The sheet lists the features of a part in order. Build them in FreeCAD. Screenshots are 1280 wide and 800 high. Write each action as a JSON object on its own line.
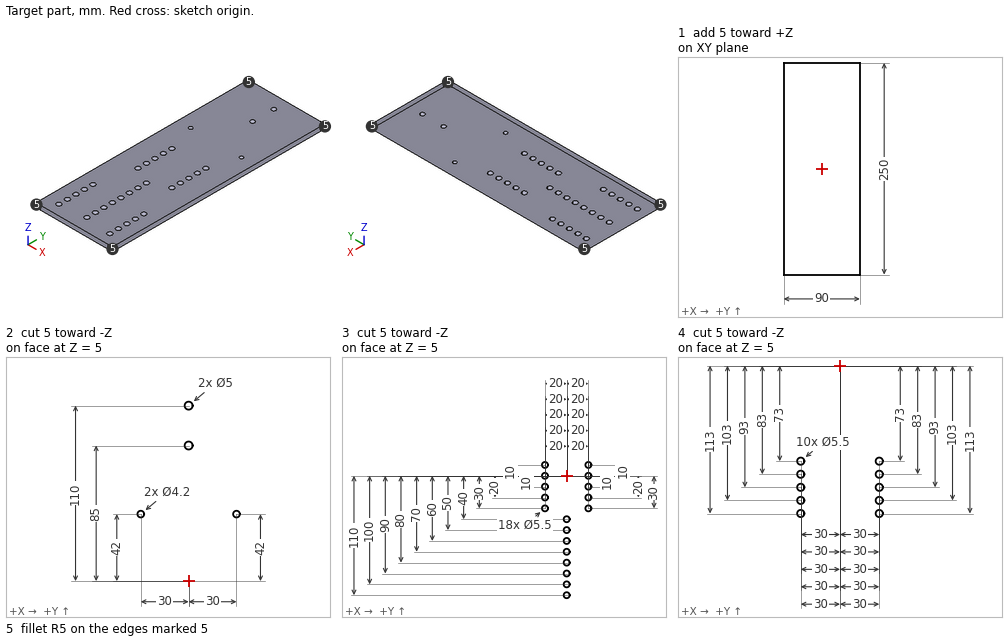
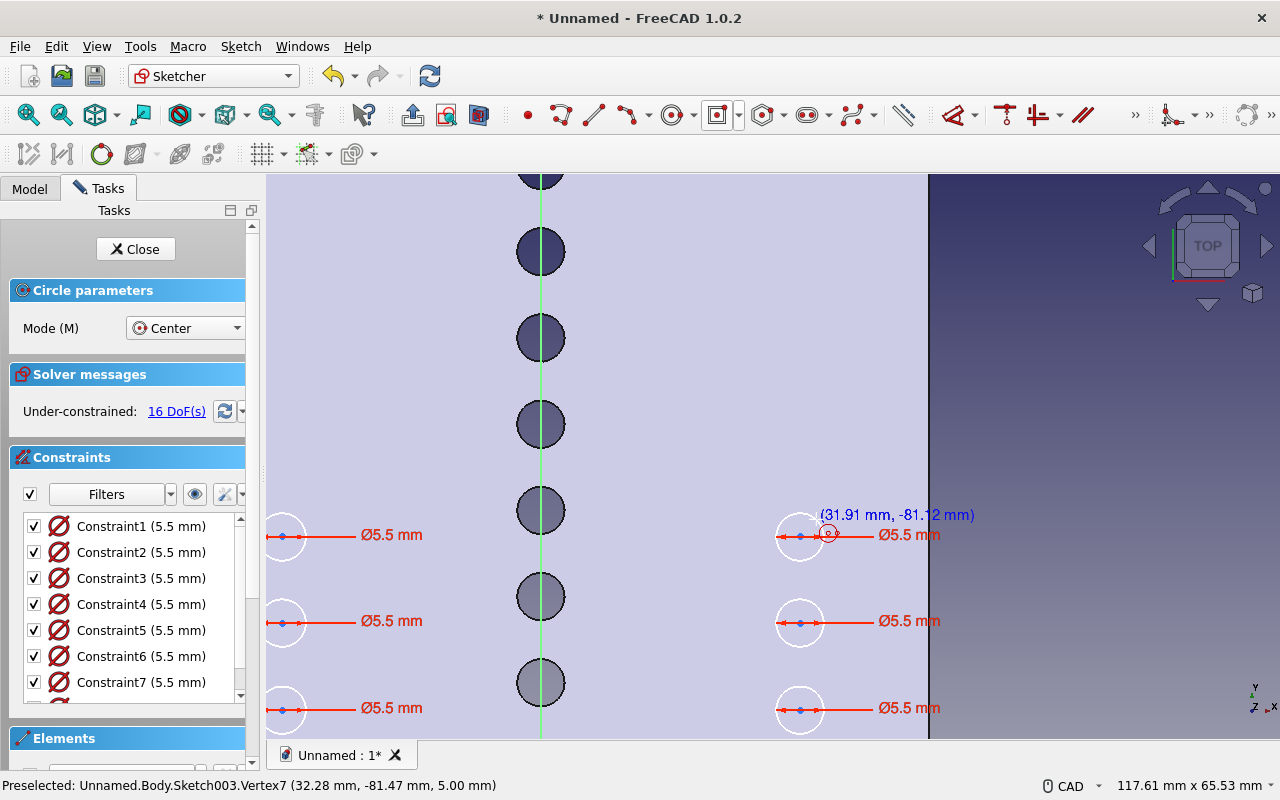
{"action": "scroll", "coordinate": [800, 536], "scroll_direction": "down", "scroll_amount": 5}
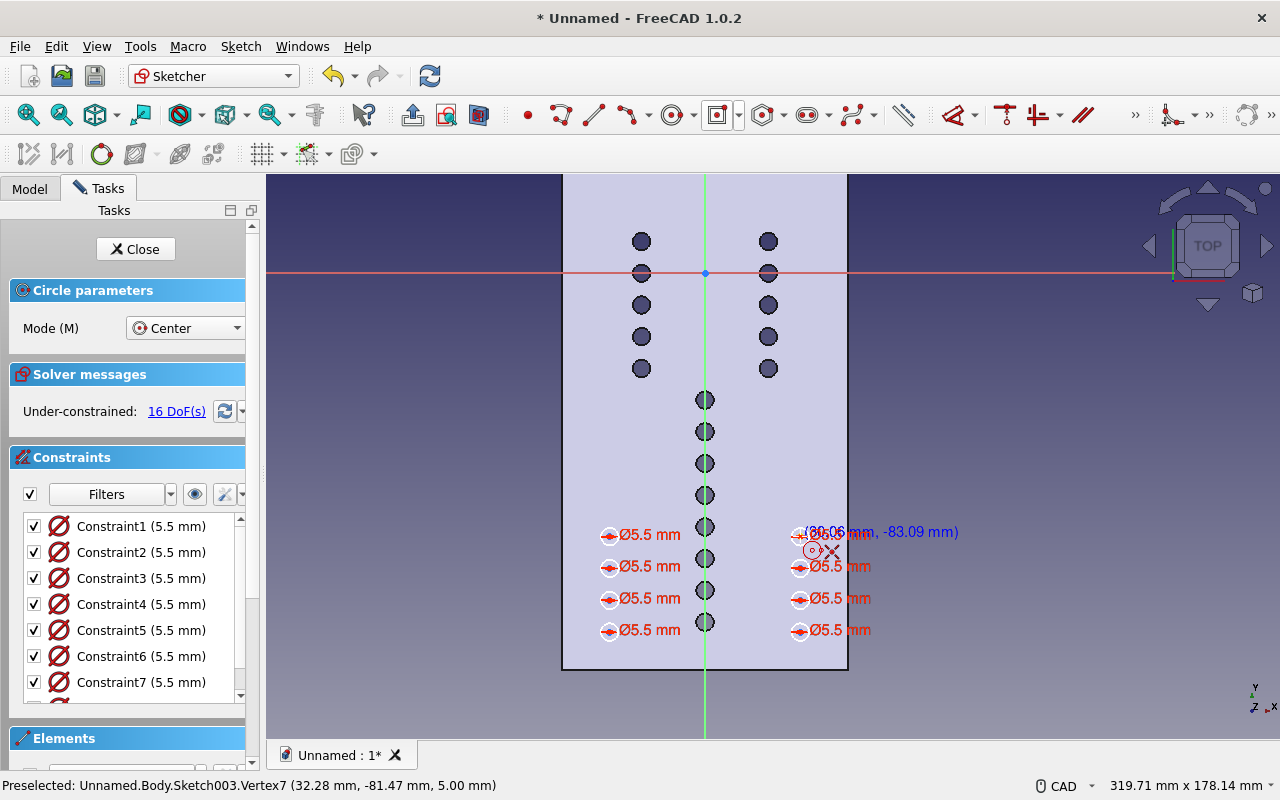
{"action": "scroll", "coordinate": [610, 505], "scroll_direction": "up", "scroll_amount": 5}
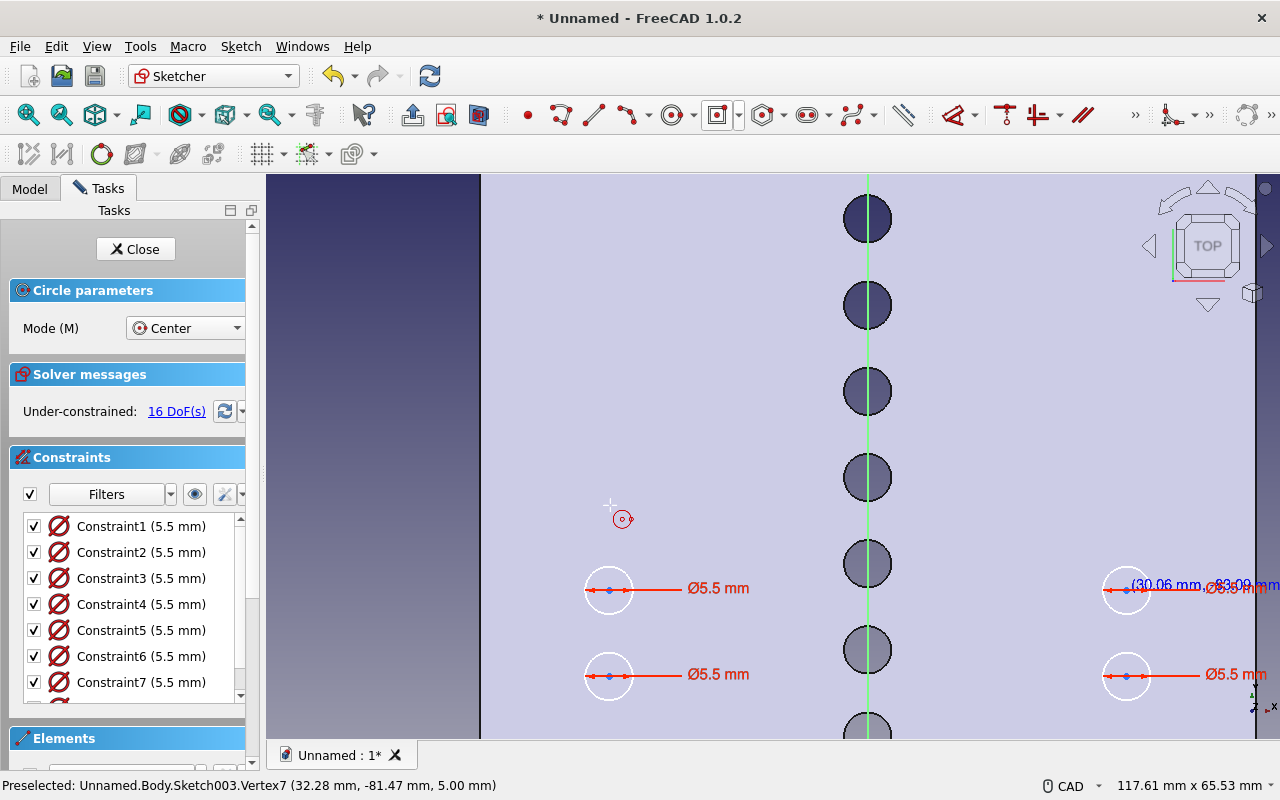
{"action": "left_click", "coordinate": [609, 503]}
{"action": "mouse_move", "coordinate": [626, 487]}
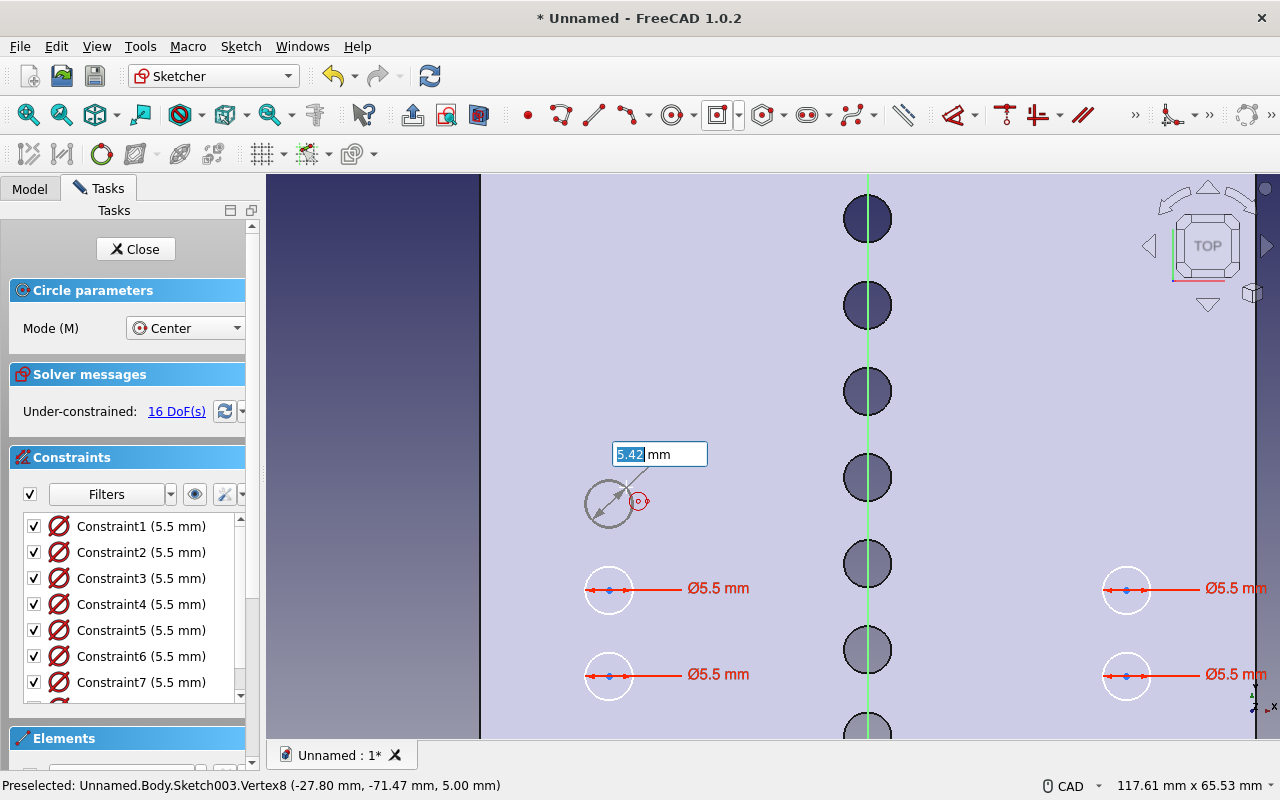
{"action": "type", "text": "5.5"}
{"action": "key", "text": "Return"}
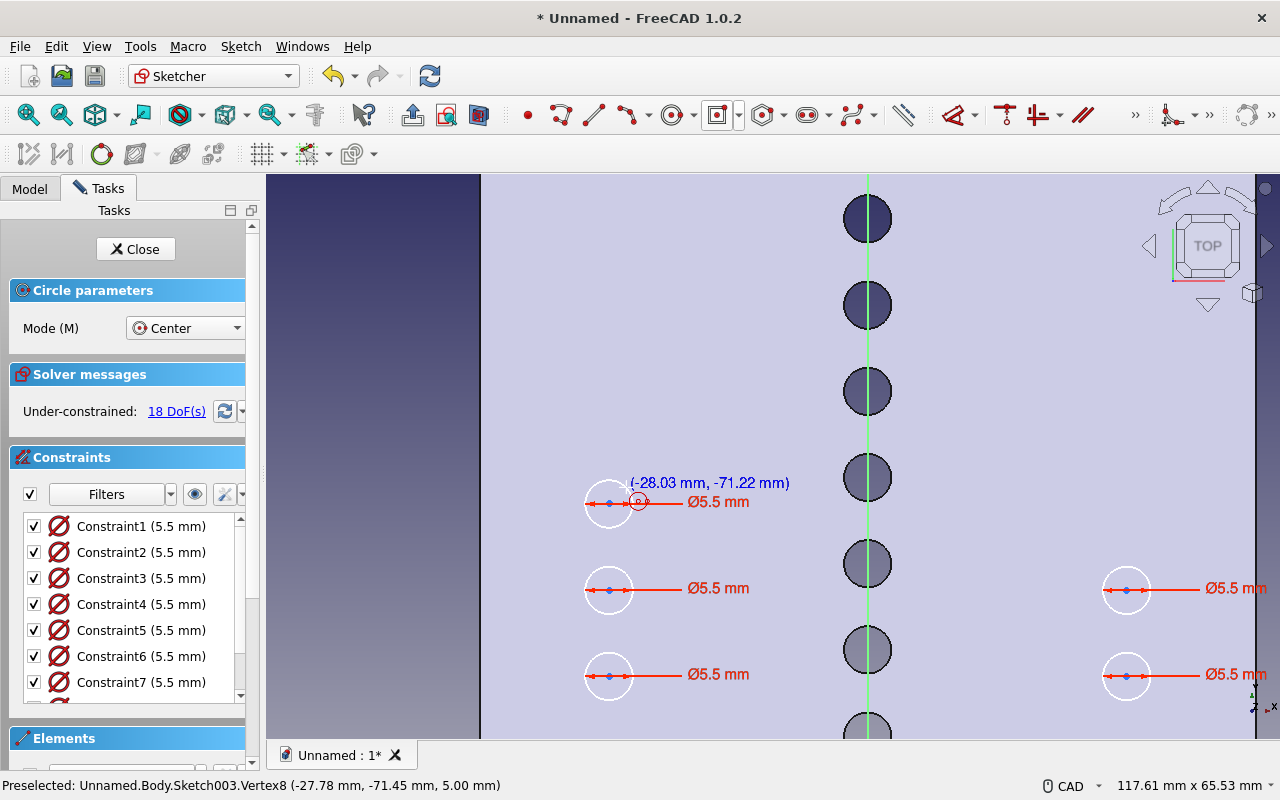
{"action": "scroll", "coordinate": [610, 505], "scroll_direction": "down", "scroll_amount": 5}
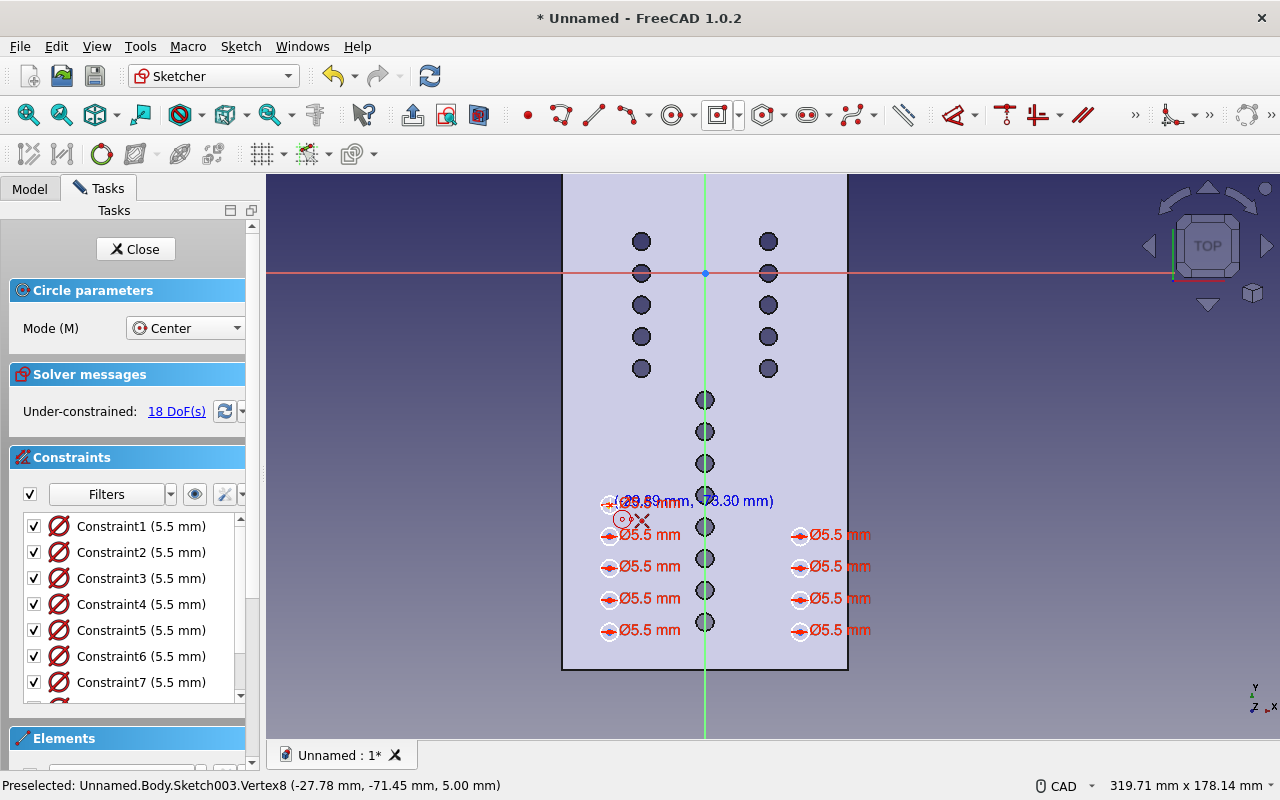
{"action": "scroll", "coordinate": [800, 505], "scroll_direction": "up", "scroll_amount": 5}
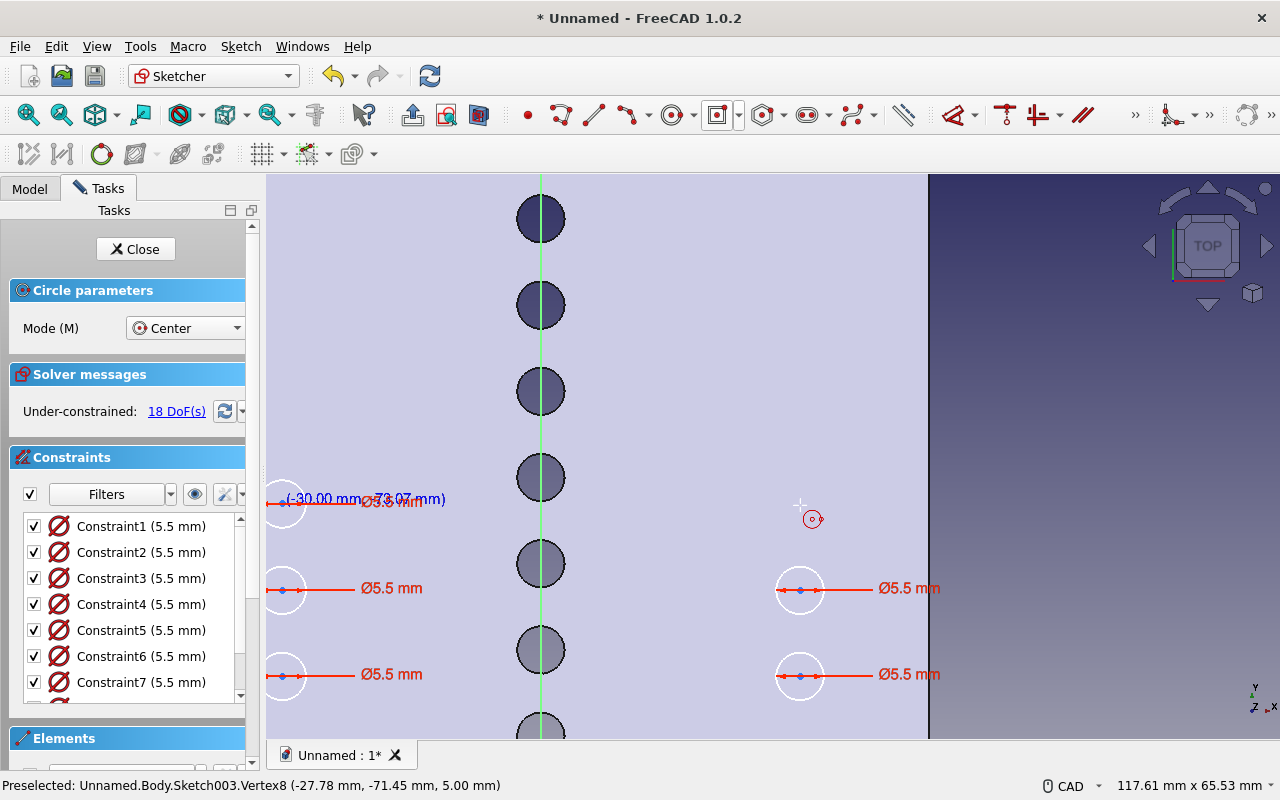
{"action": "left_click", "coordinate": [800, 503]}
{"action": "mouse_move", "coordinate": [816, 487]}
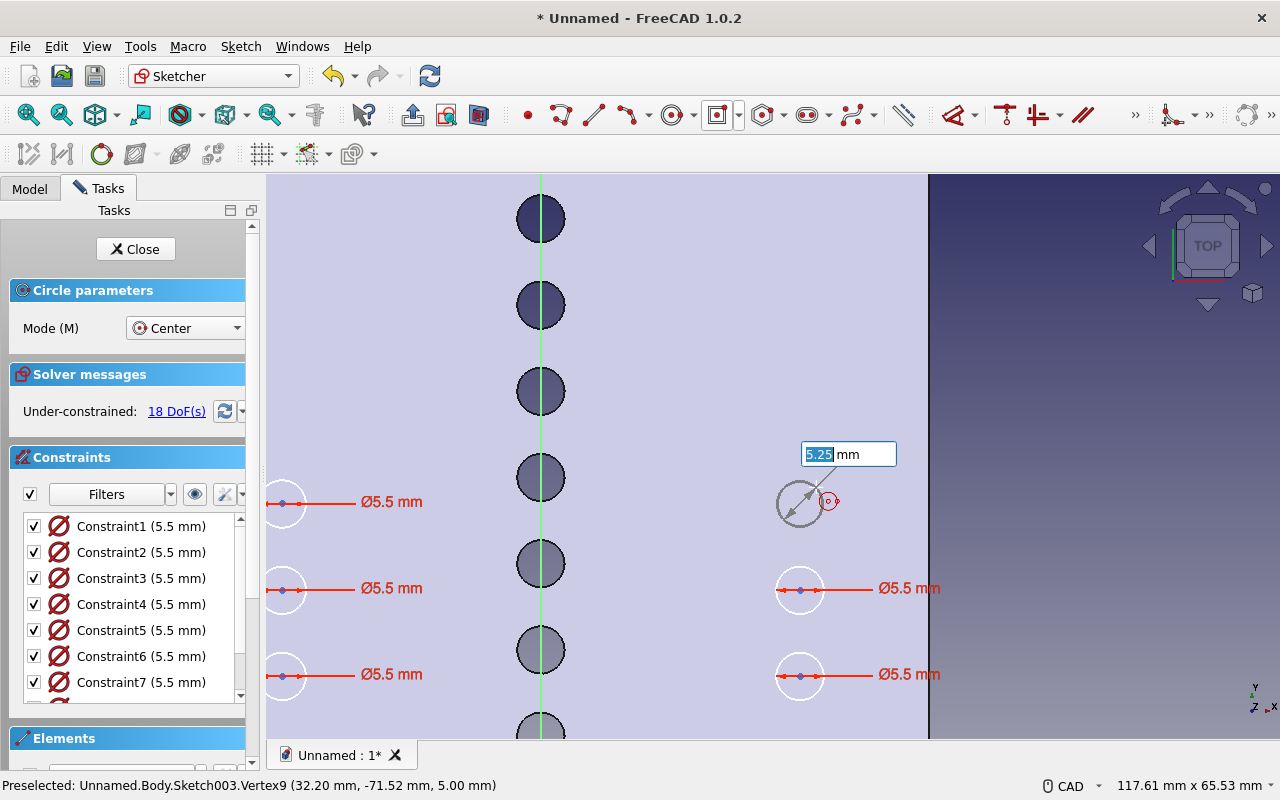
{"action": "type", "text": "5.5"}
{"action": "key", "text": "Return"}
{"action": "key", "text": "Escape"}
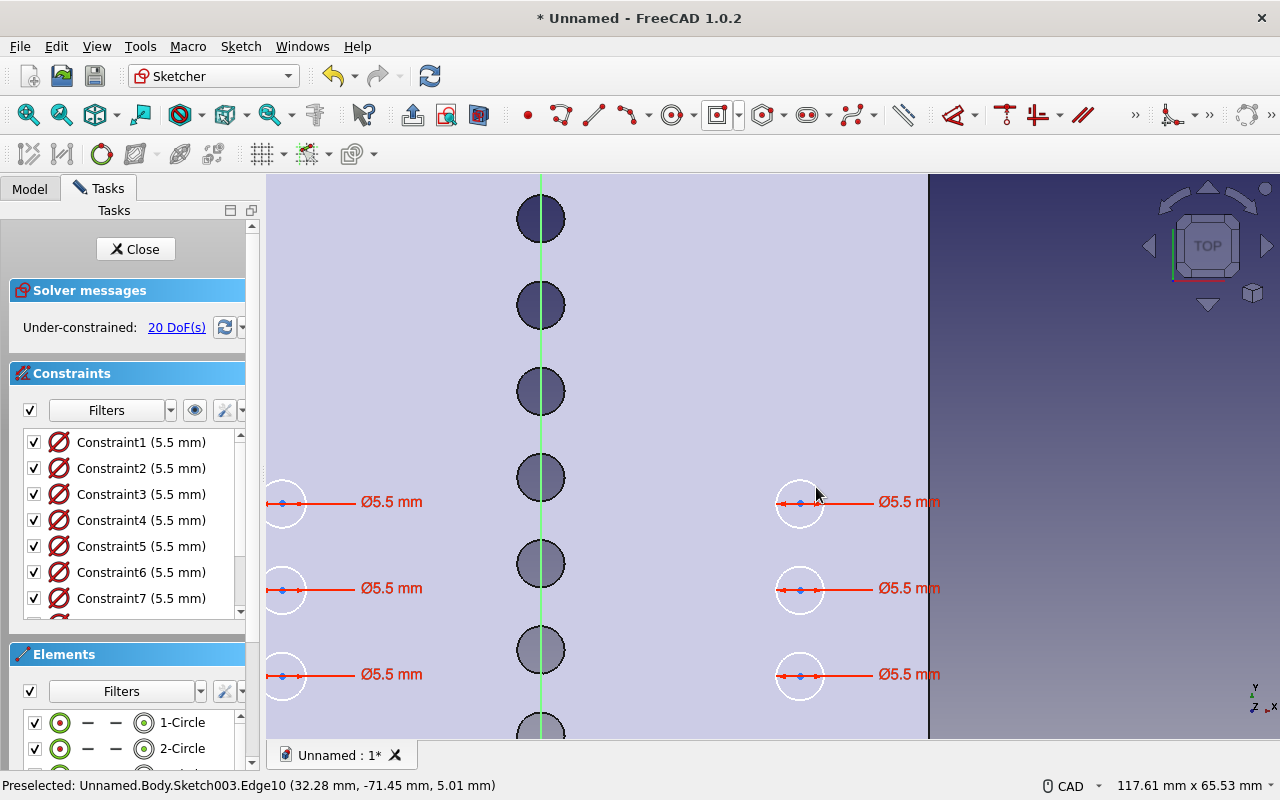
{"action": "key", "text": "d"}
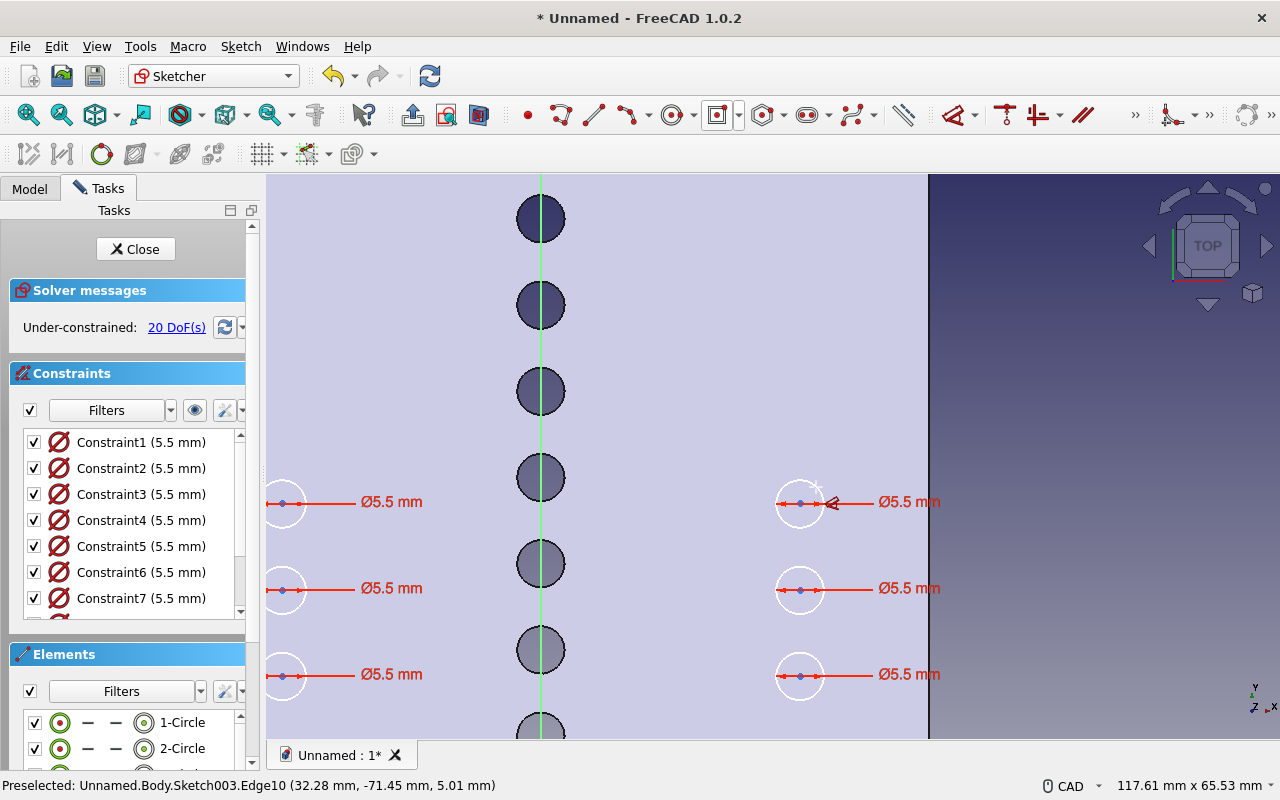
{"action": "scroll", "coordinate": [800, 505], "scroll_direction": "down", "scroll_amount": 5}